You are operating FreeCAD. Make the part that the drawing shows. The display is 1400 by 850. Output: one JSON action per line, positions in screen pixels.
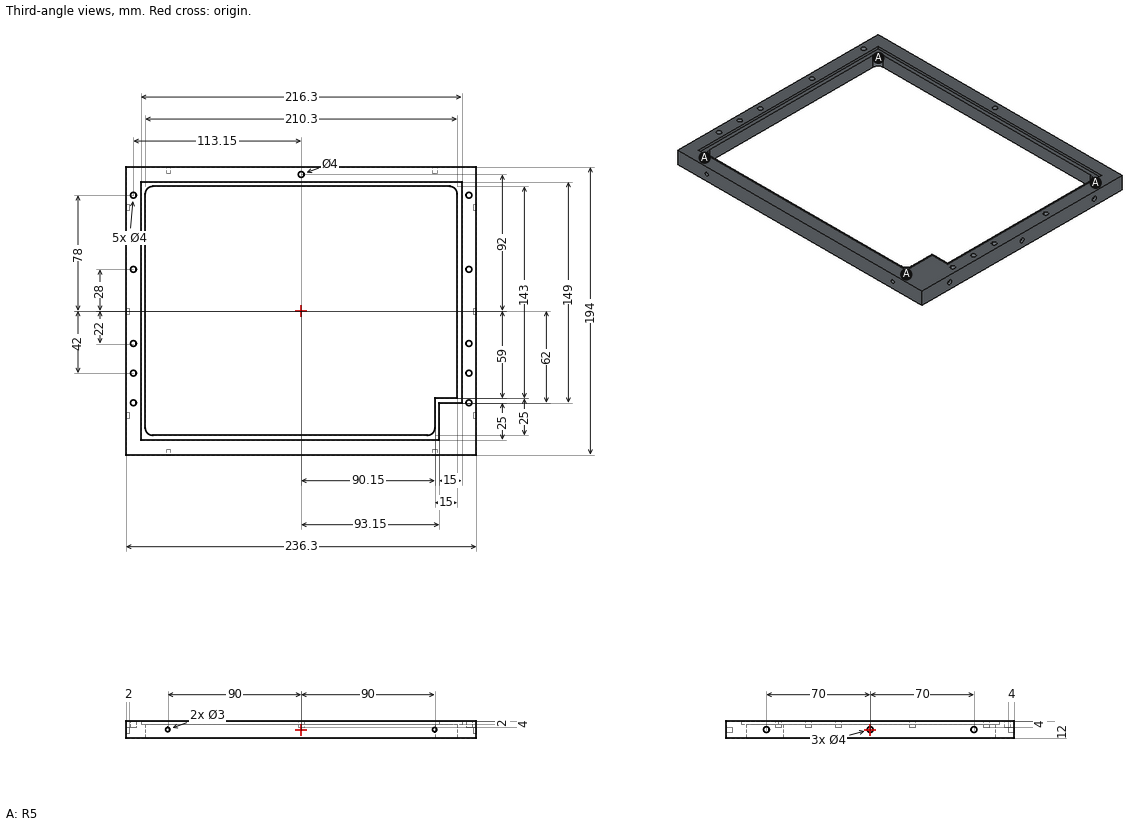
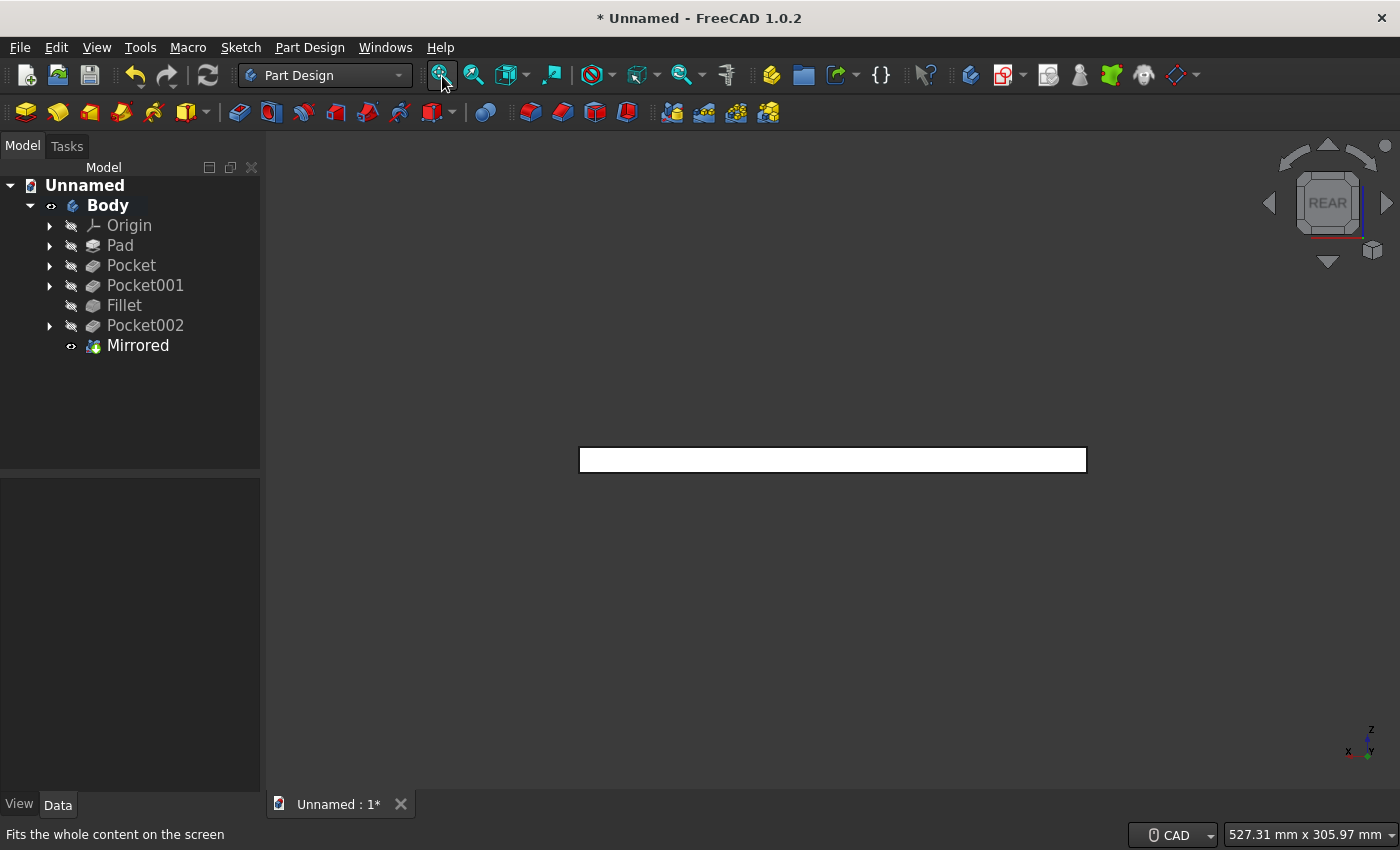
{"action": "left_click", "coordinate": [442, 76]}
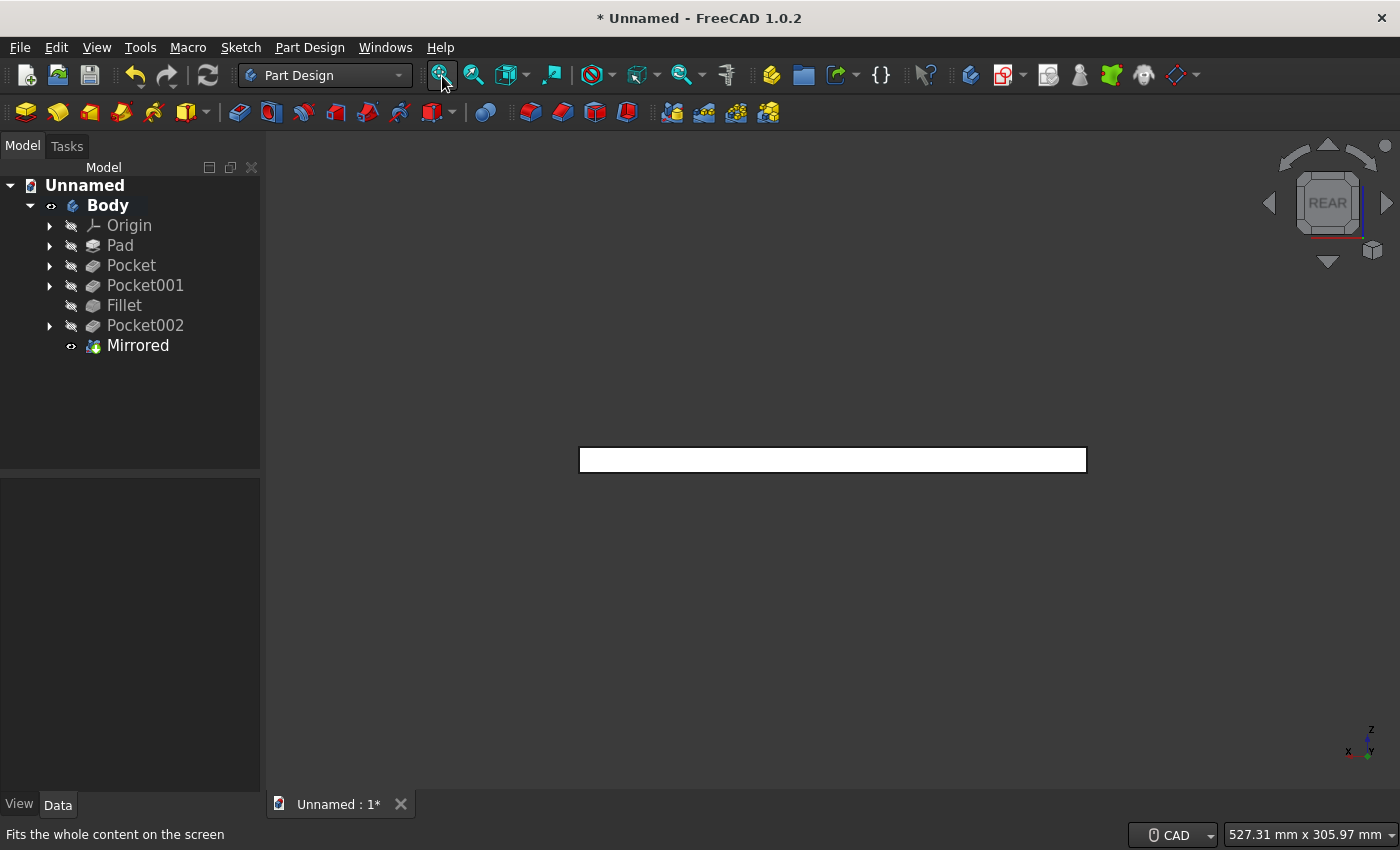
{"action": "left_click", "coordinate": [615, 459]}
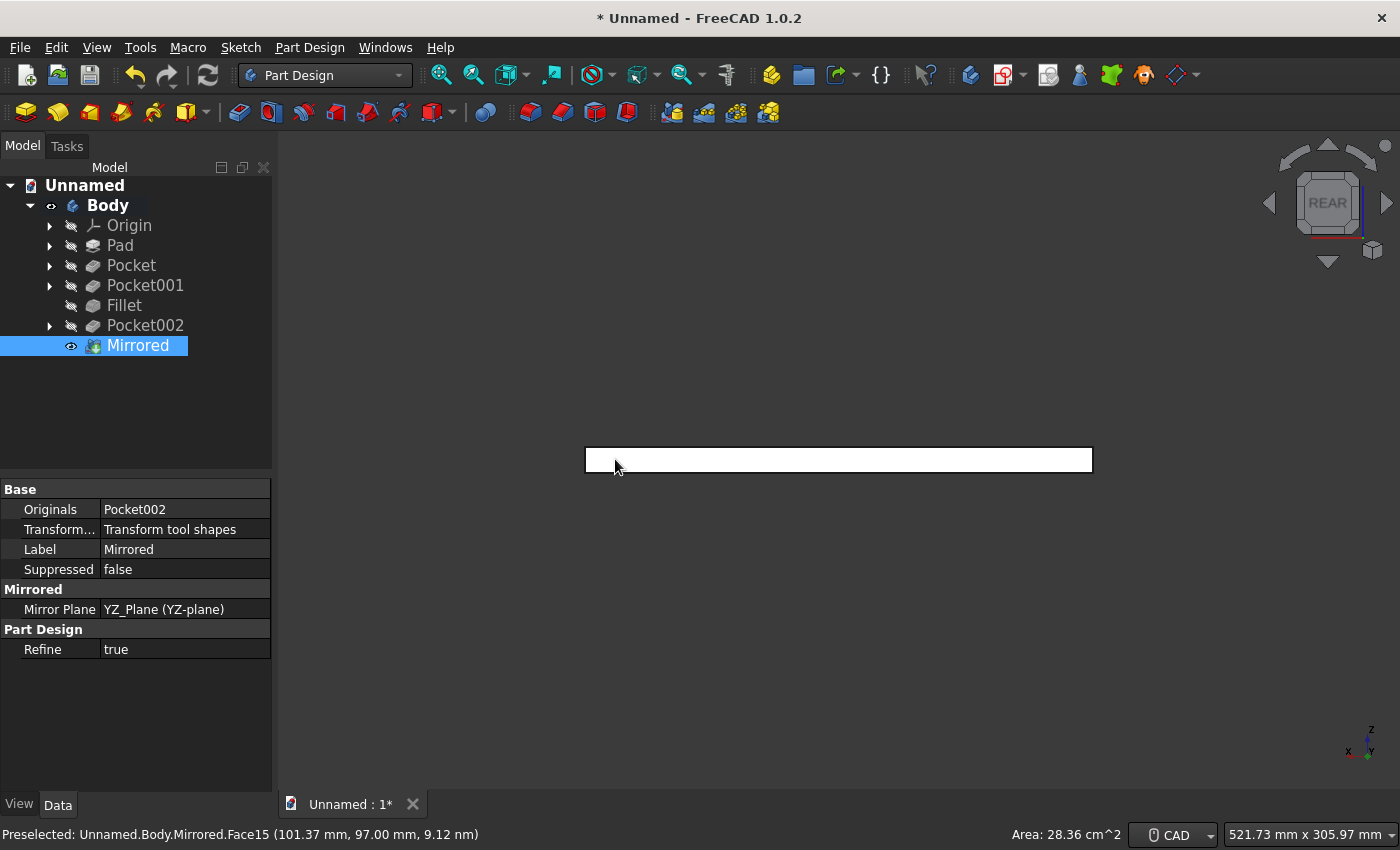
{"action": "left_click", "coordinate": [1004, 76]}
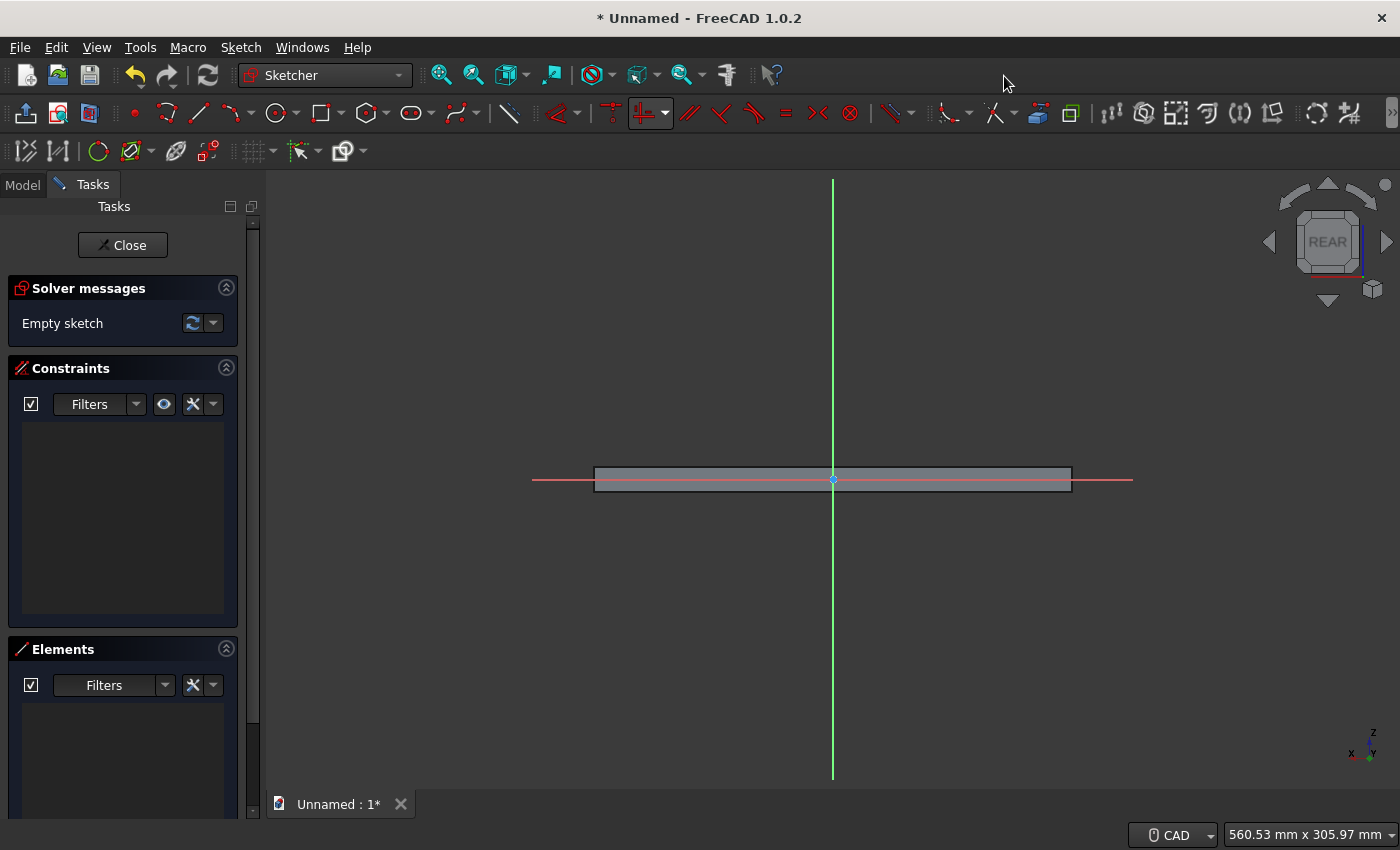
{"action": "scroll", "coordinate": [916, 480], "scroll_direction": "up", "scroll_amount": 3}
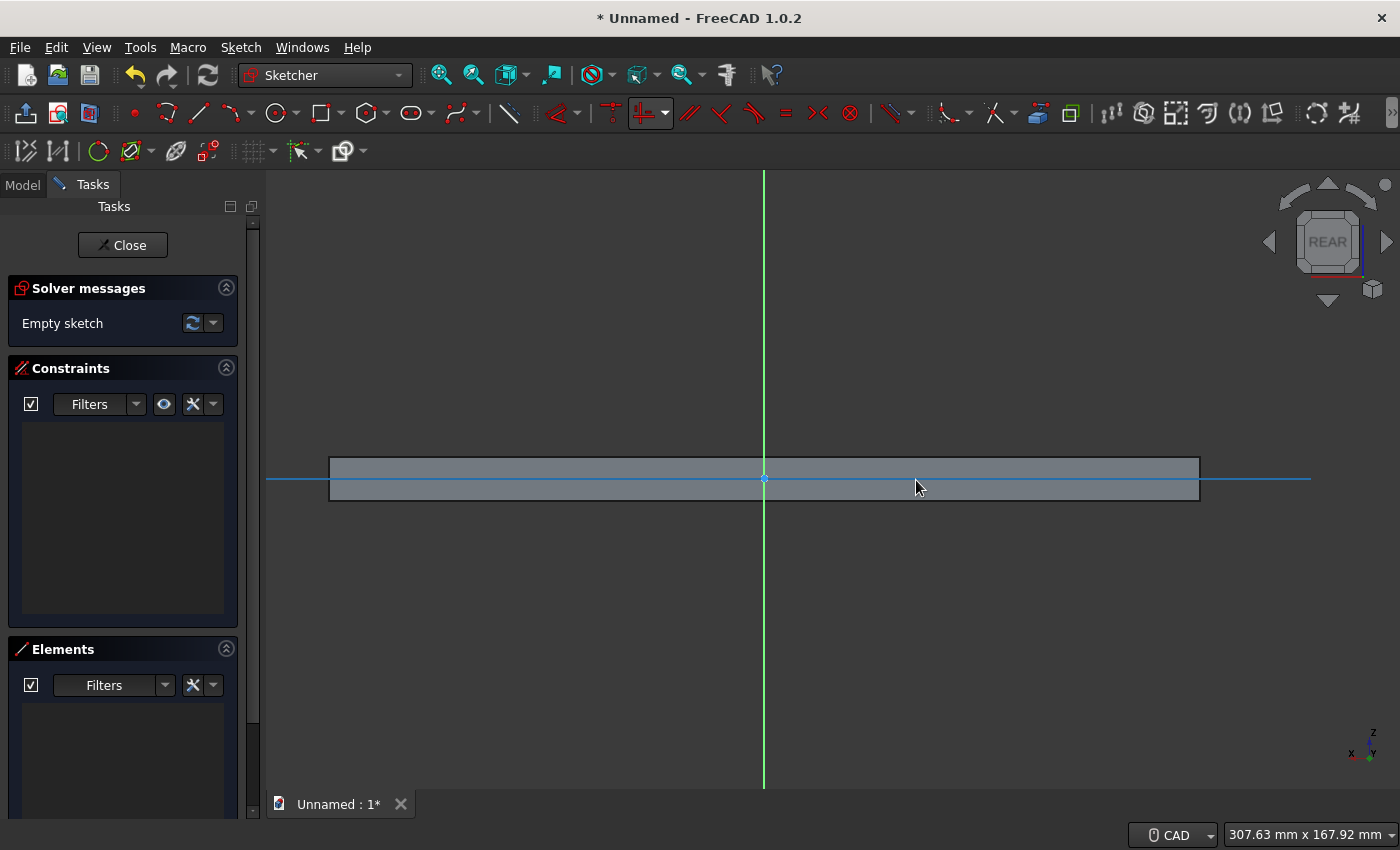
{"action": "left_click", "coordinate": [276, 114]}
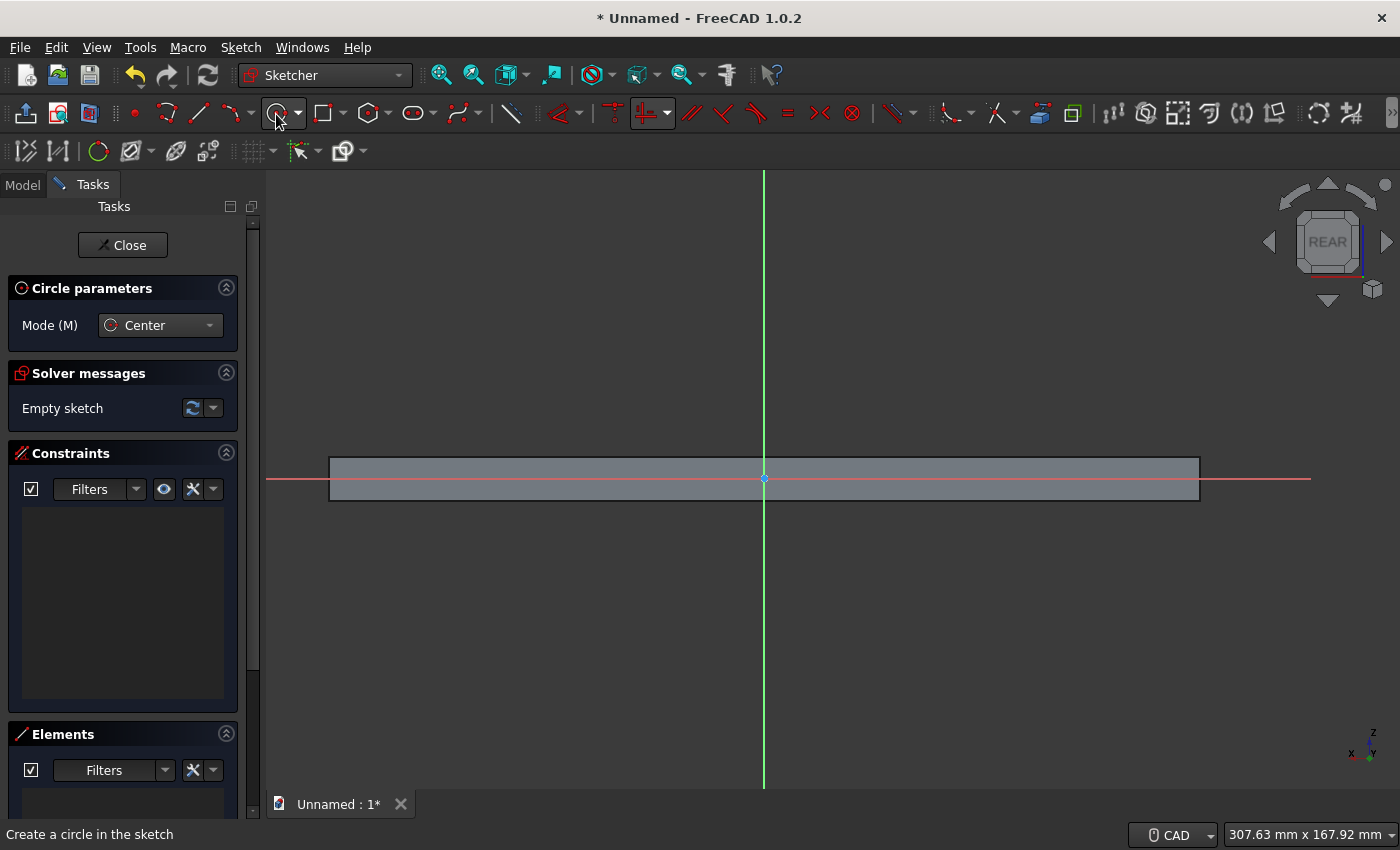
{"action": "scroll", "coordinate": [1096, 479], "scroll_direction": "up", "scroll_amount": 8}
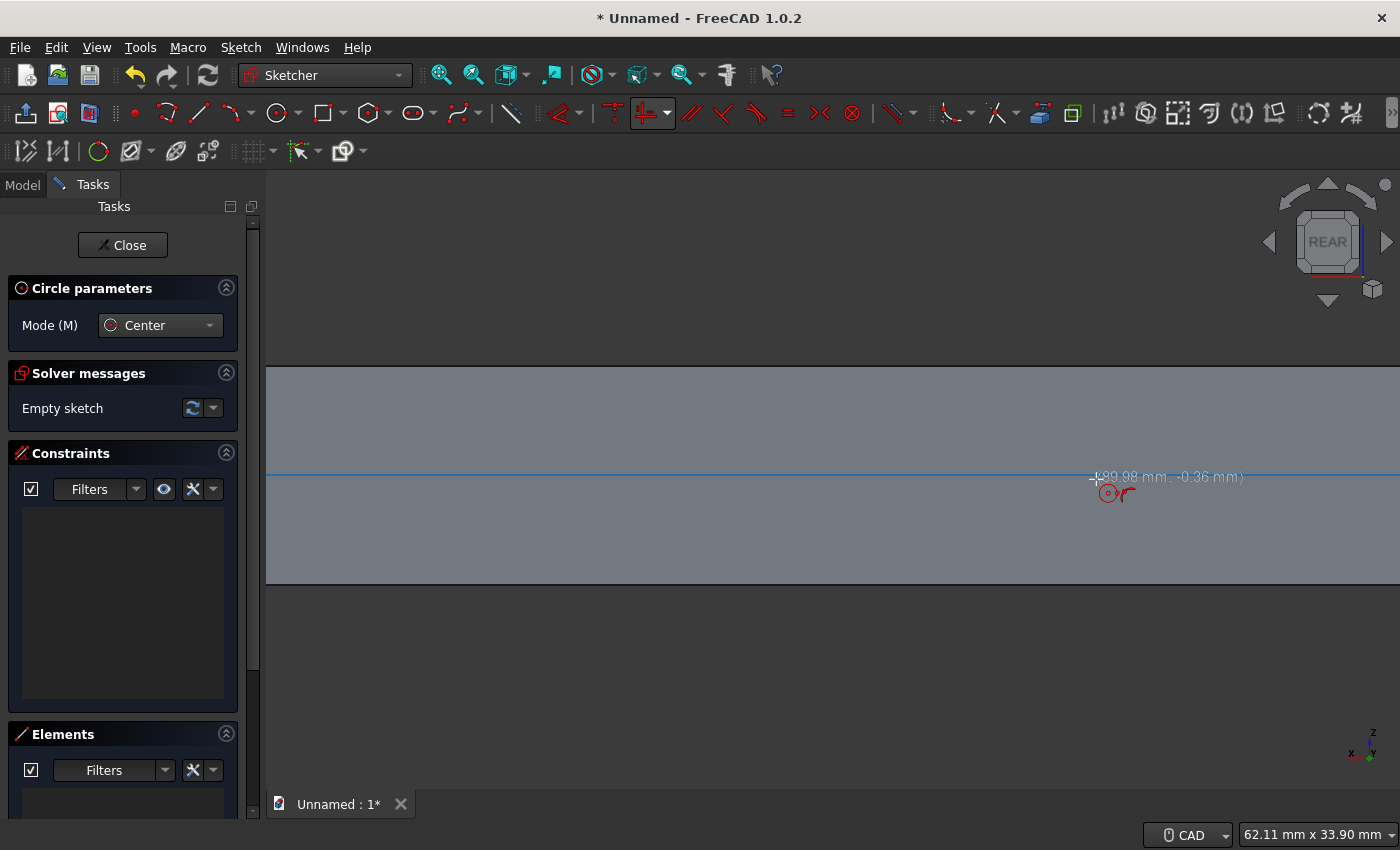
{"action": "scroll", "coordinate": [1097, 481], "scroll_direction": "down", "scroll_amount": 8}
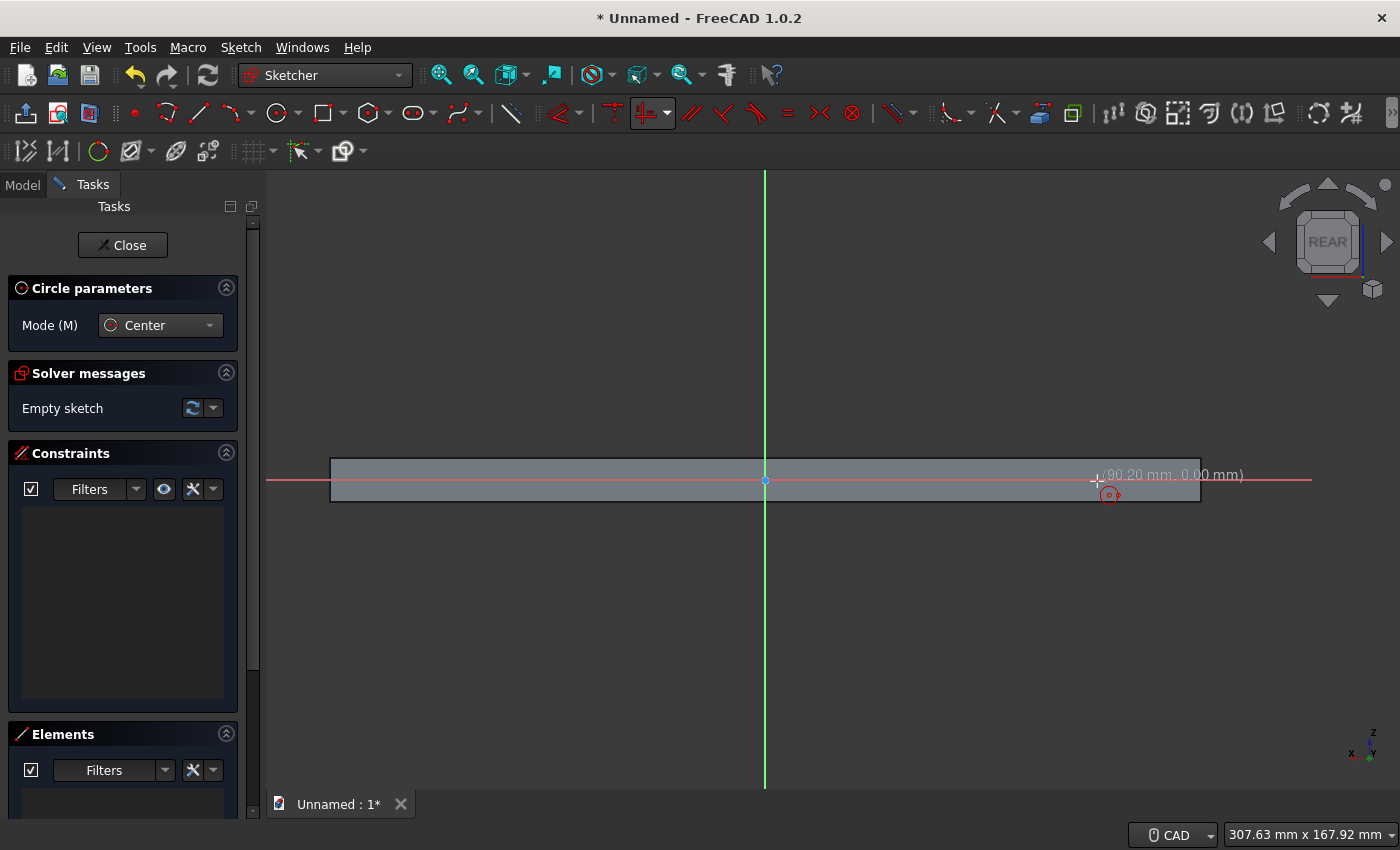
{"action": "left_click", "coordinate": [1097, 480]}